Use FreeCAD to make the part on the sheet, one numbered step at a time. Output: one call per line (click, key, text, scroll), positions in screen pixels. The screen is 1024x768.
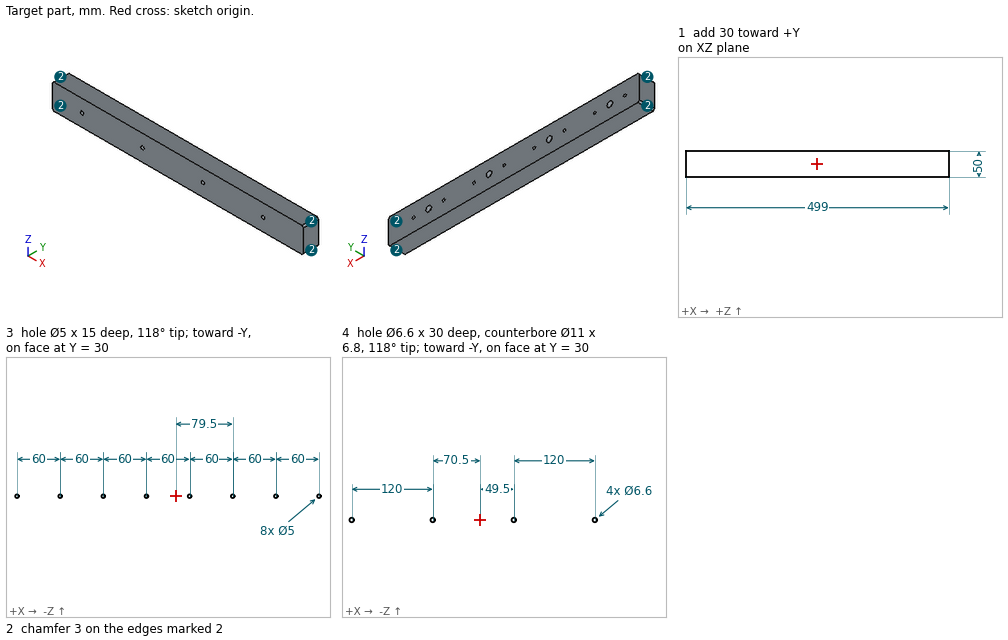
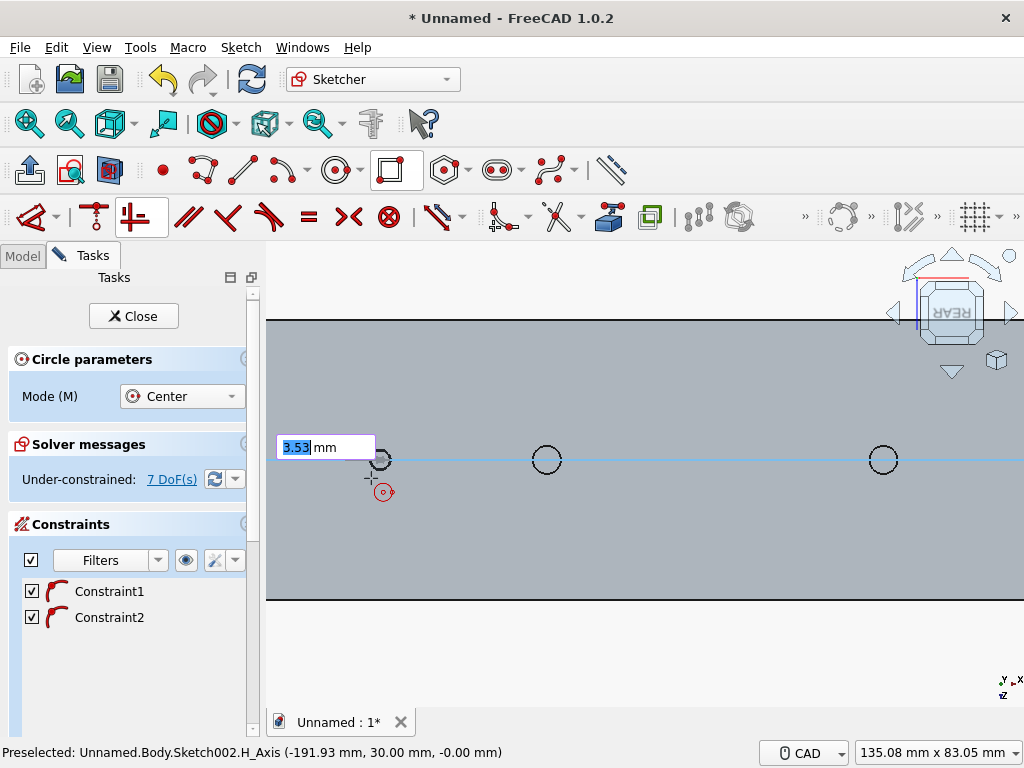
click(372, 477)
key(Escape)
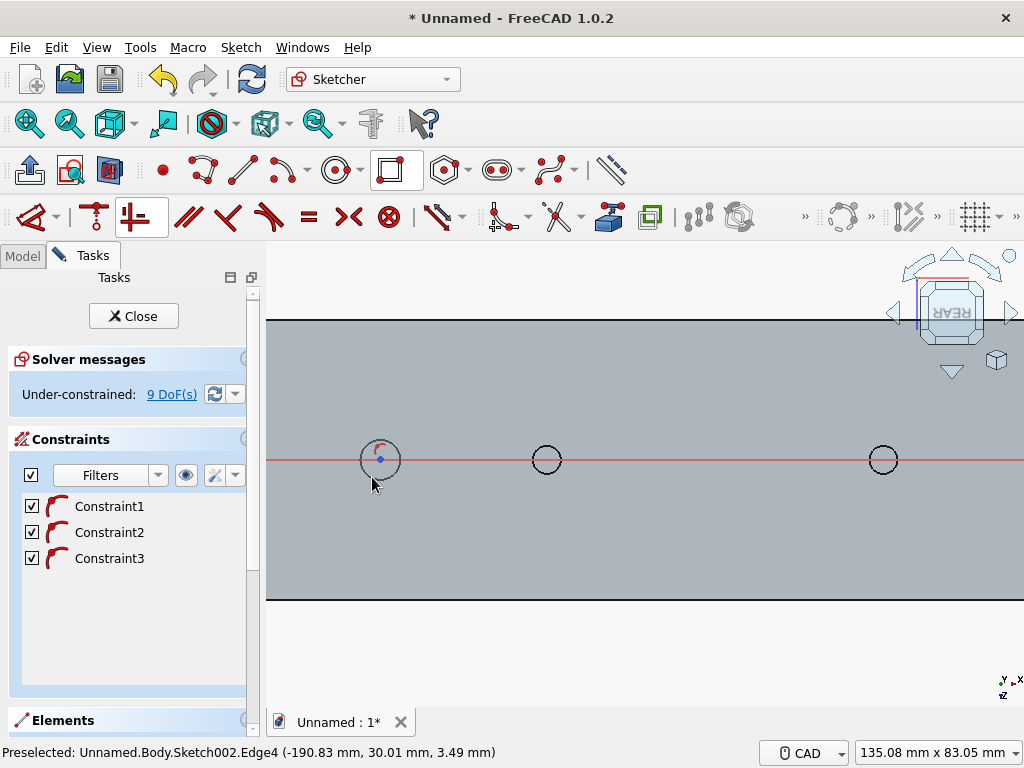
scroll(371, 478, down, 8)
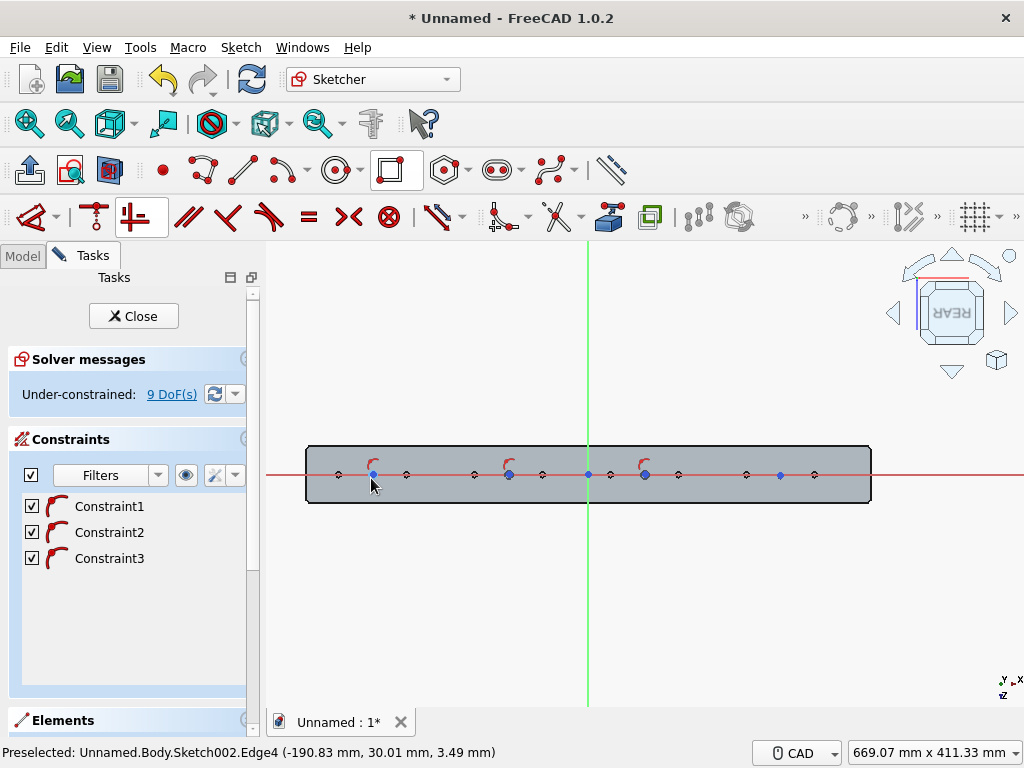
scroll(782, 474, up, 9)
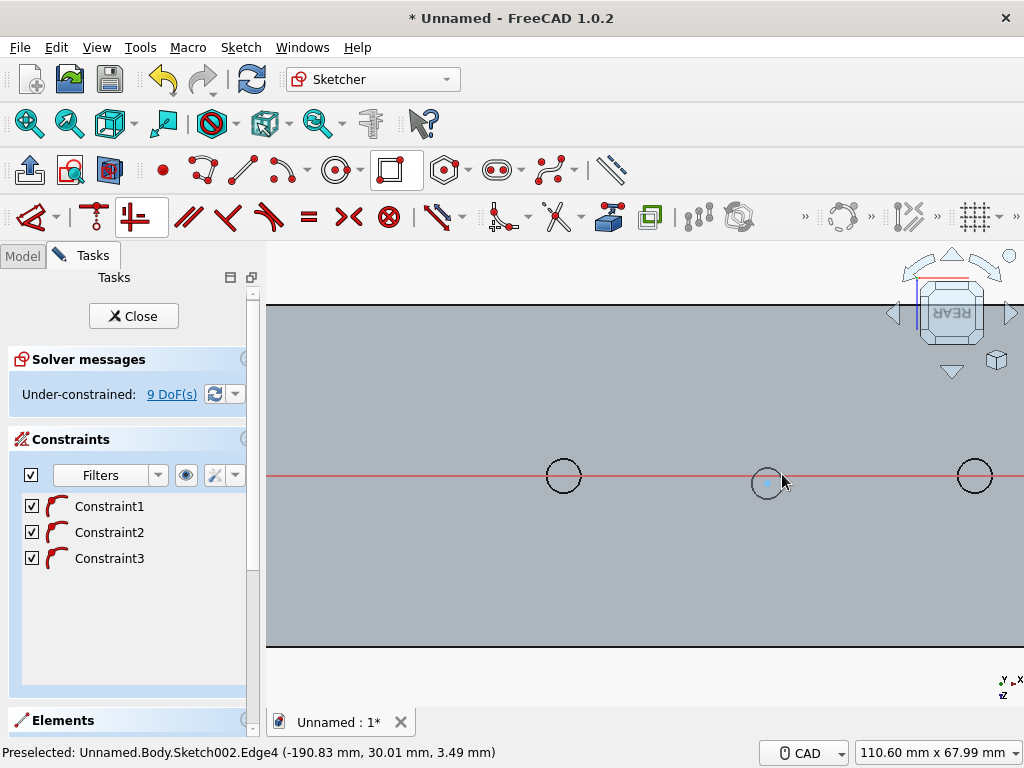
click(778, 473)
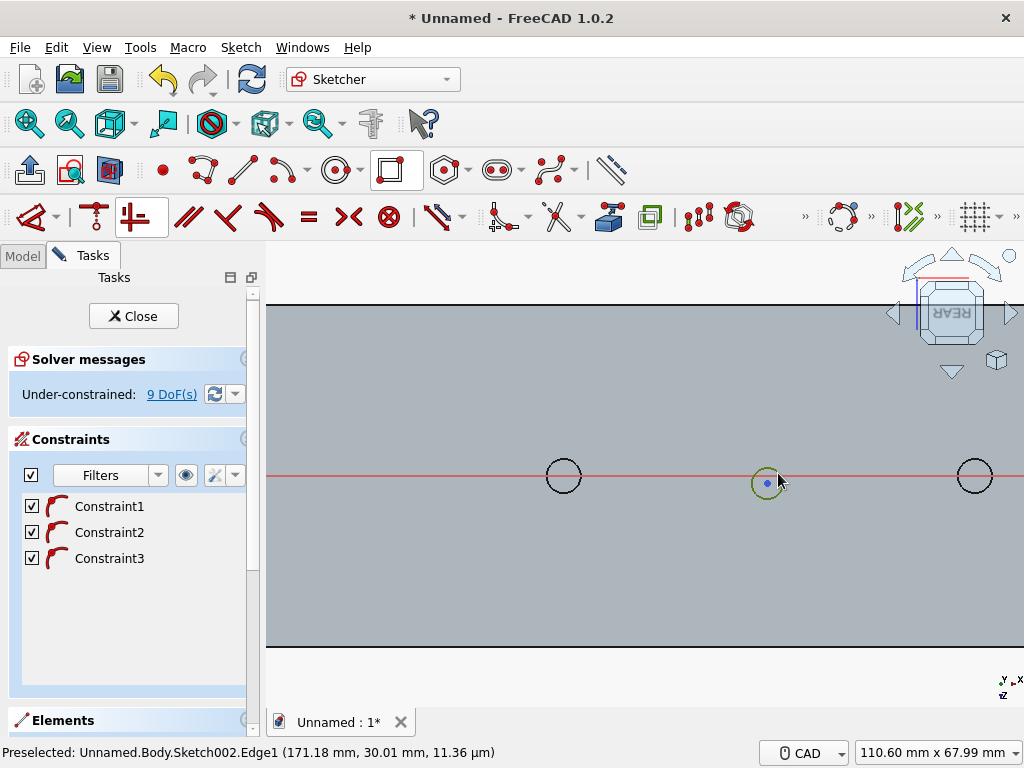
scroll(783, 474, down, 9)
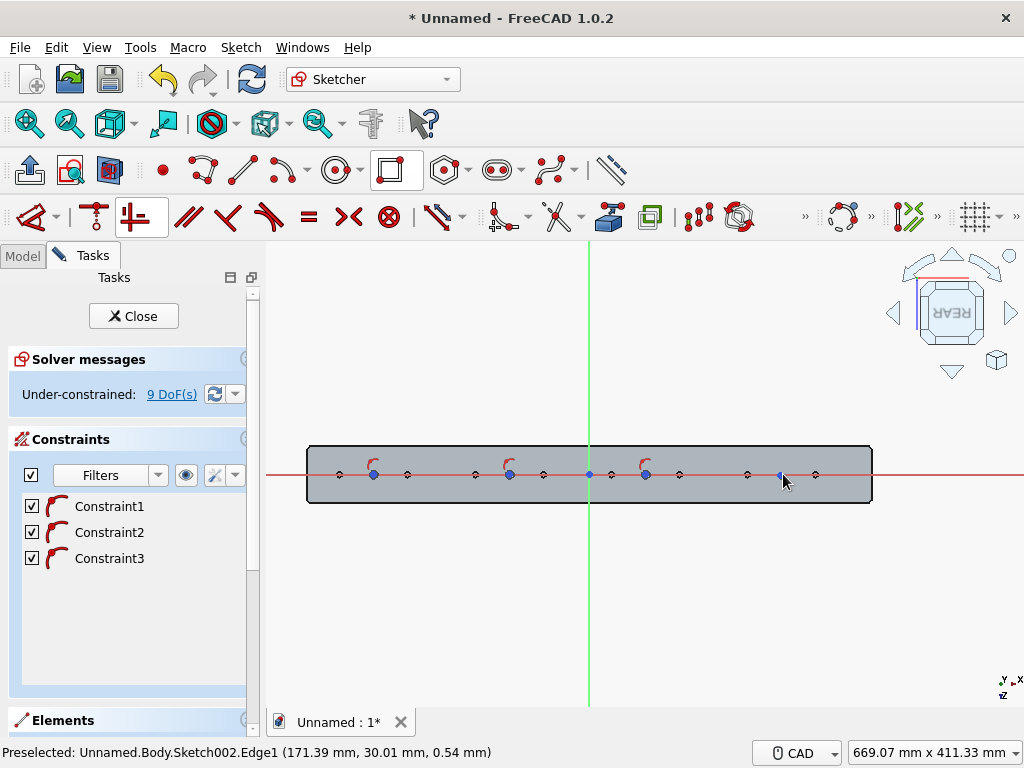
scroll(649, 472, up, 8)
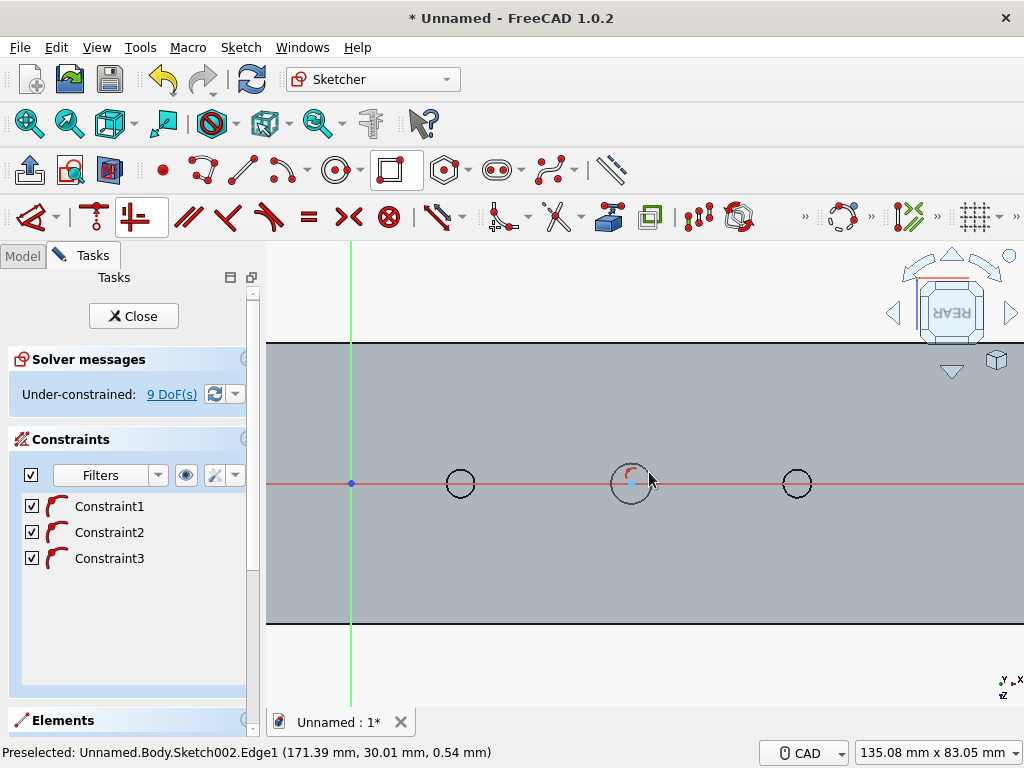
click(646, 469)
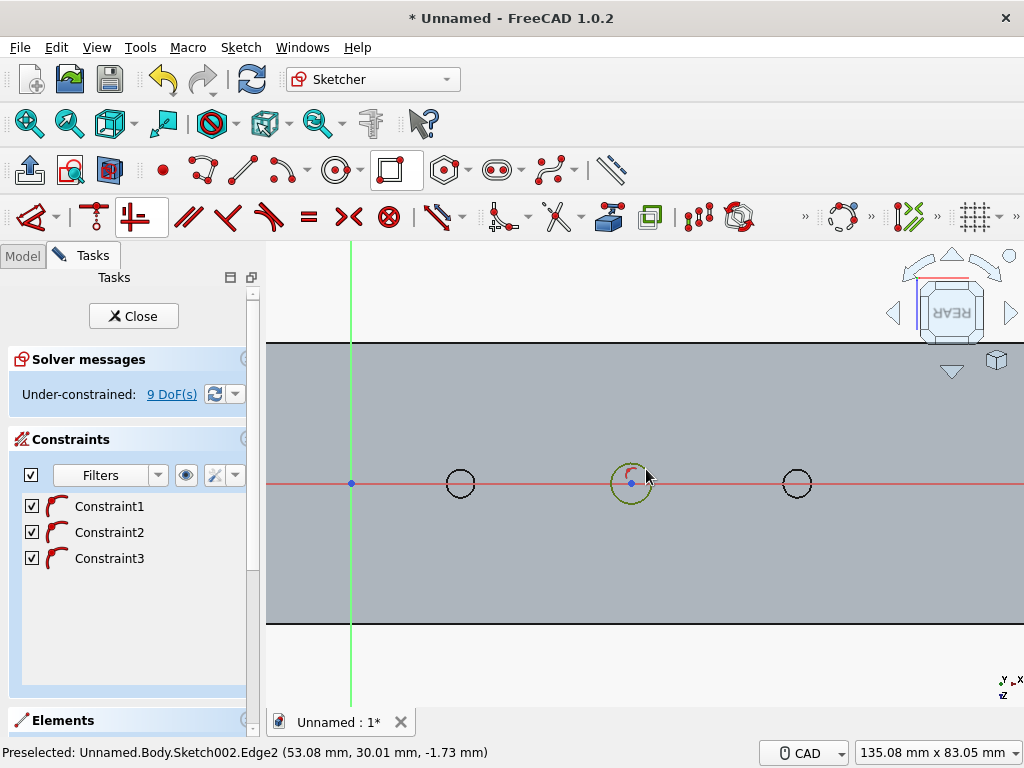
scroll(648, 472, down, 8)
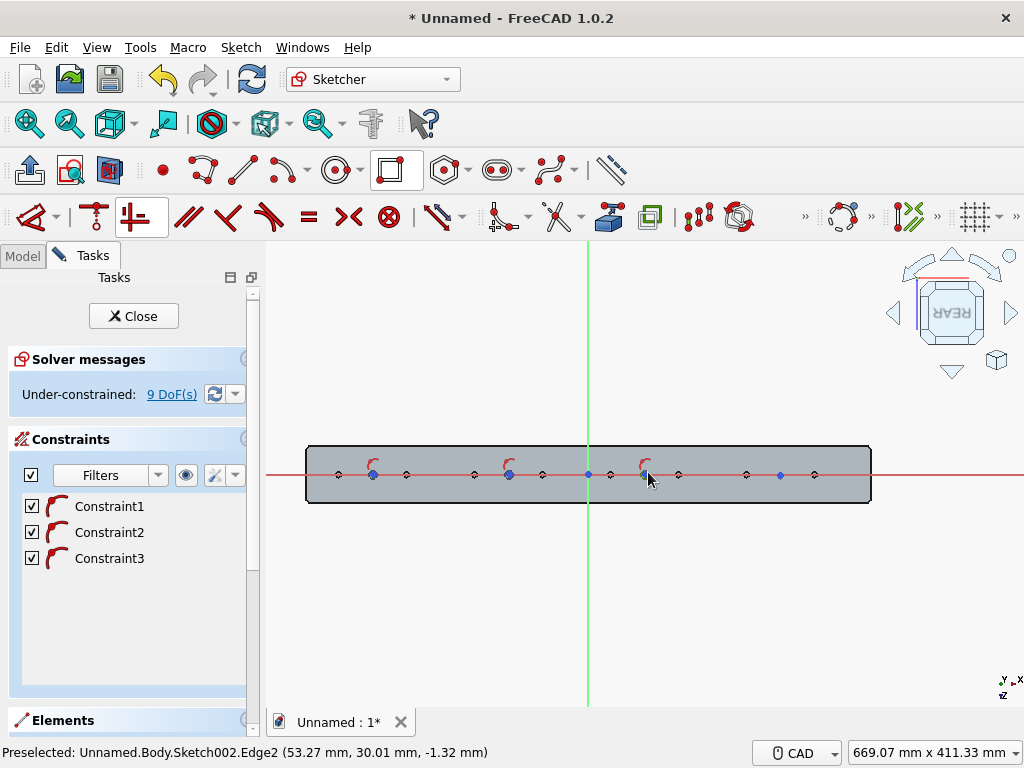
scroll(512, 472, up, 8)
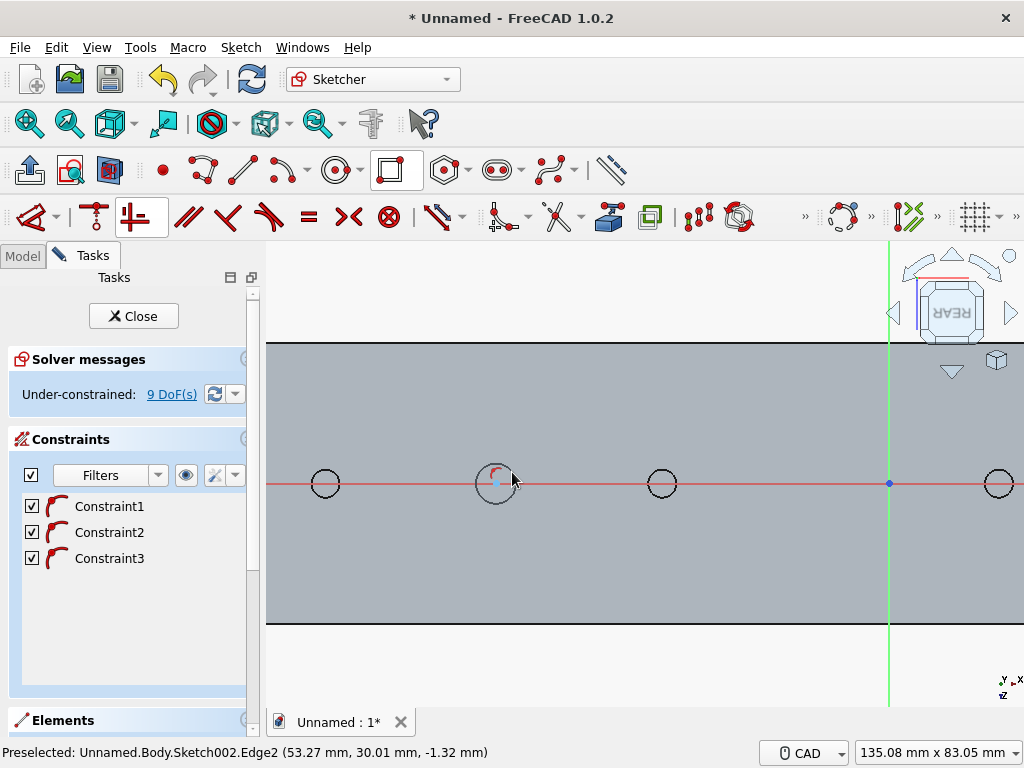
click(510, 469)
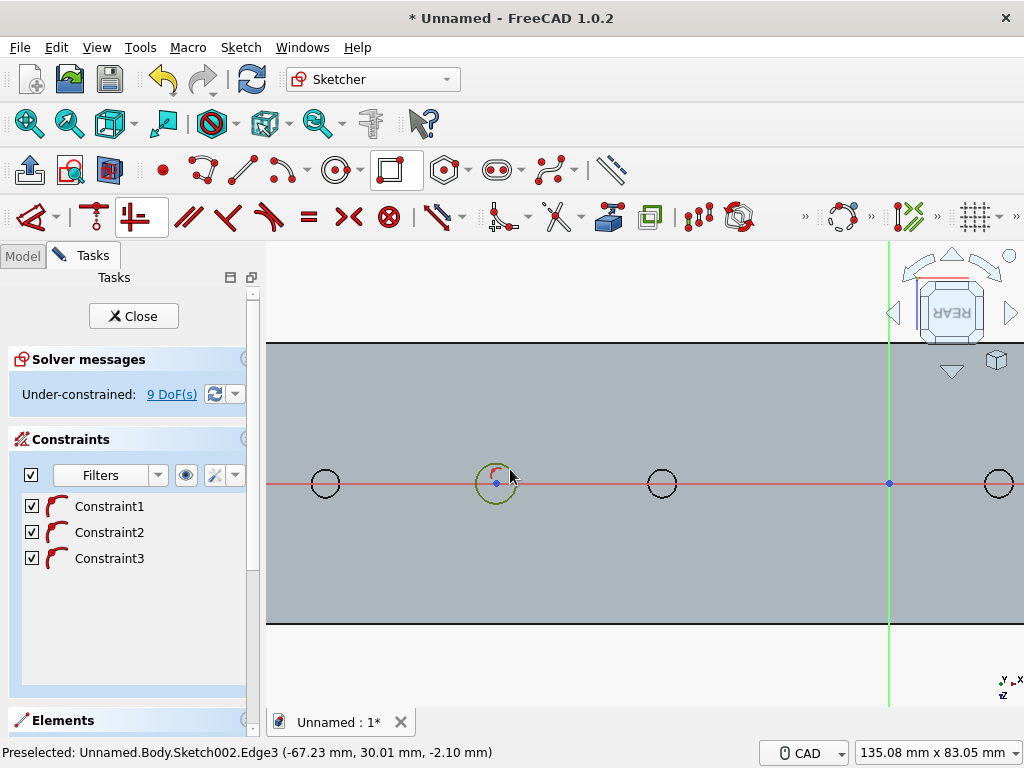
scroll(512, 472, down, 8)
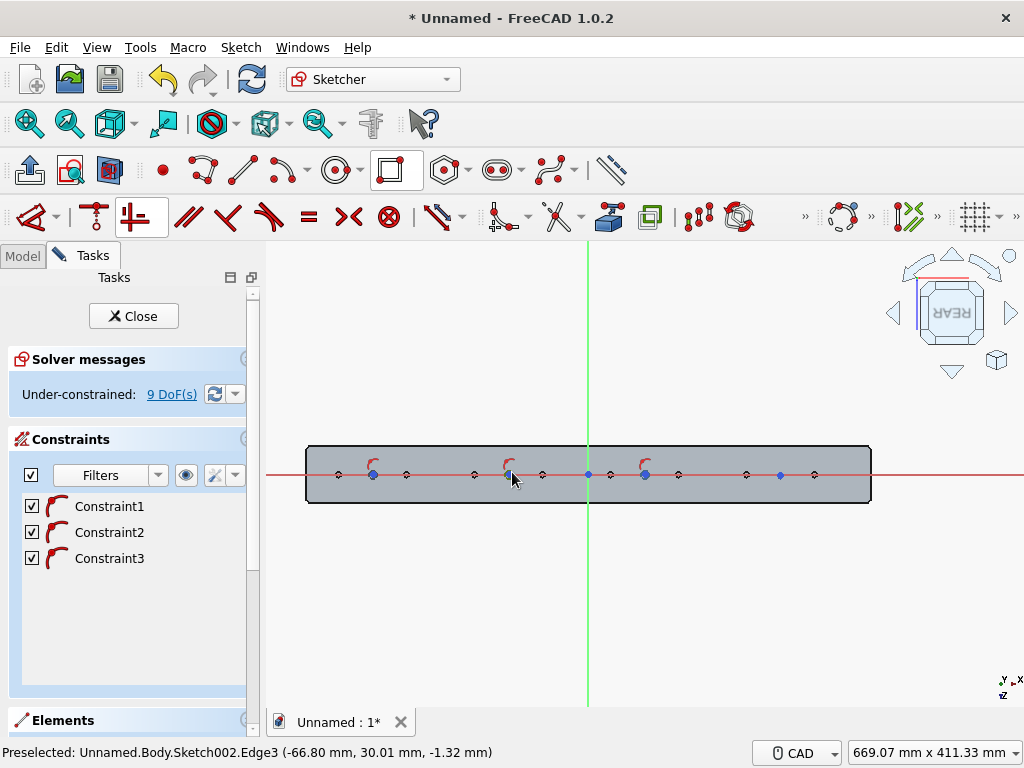
scroll(376, 472, up, 8)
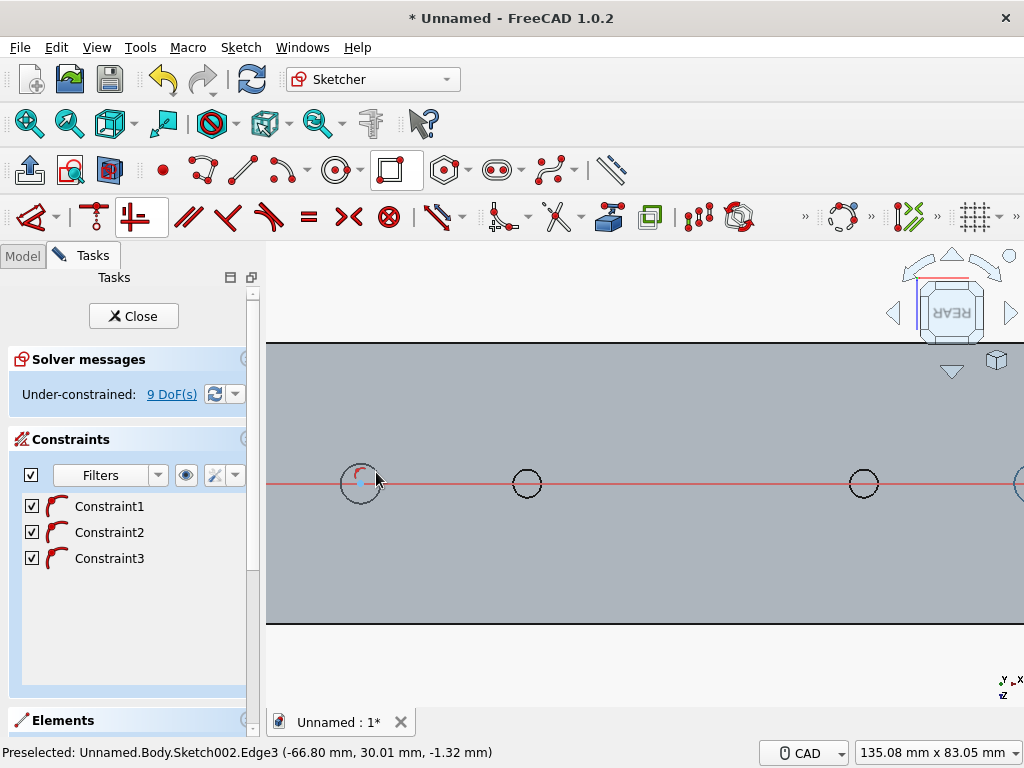
click(375, 470)